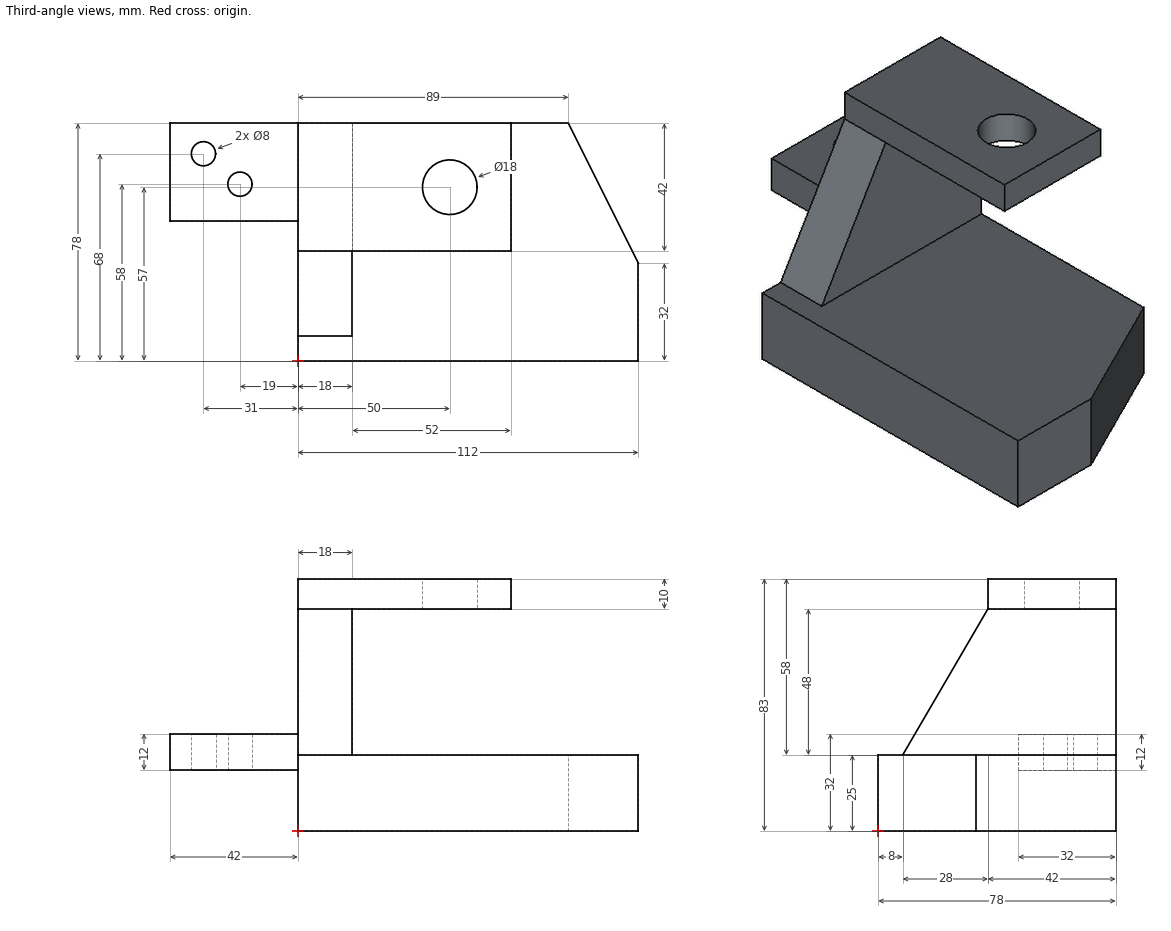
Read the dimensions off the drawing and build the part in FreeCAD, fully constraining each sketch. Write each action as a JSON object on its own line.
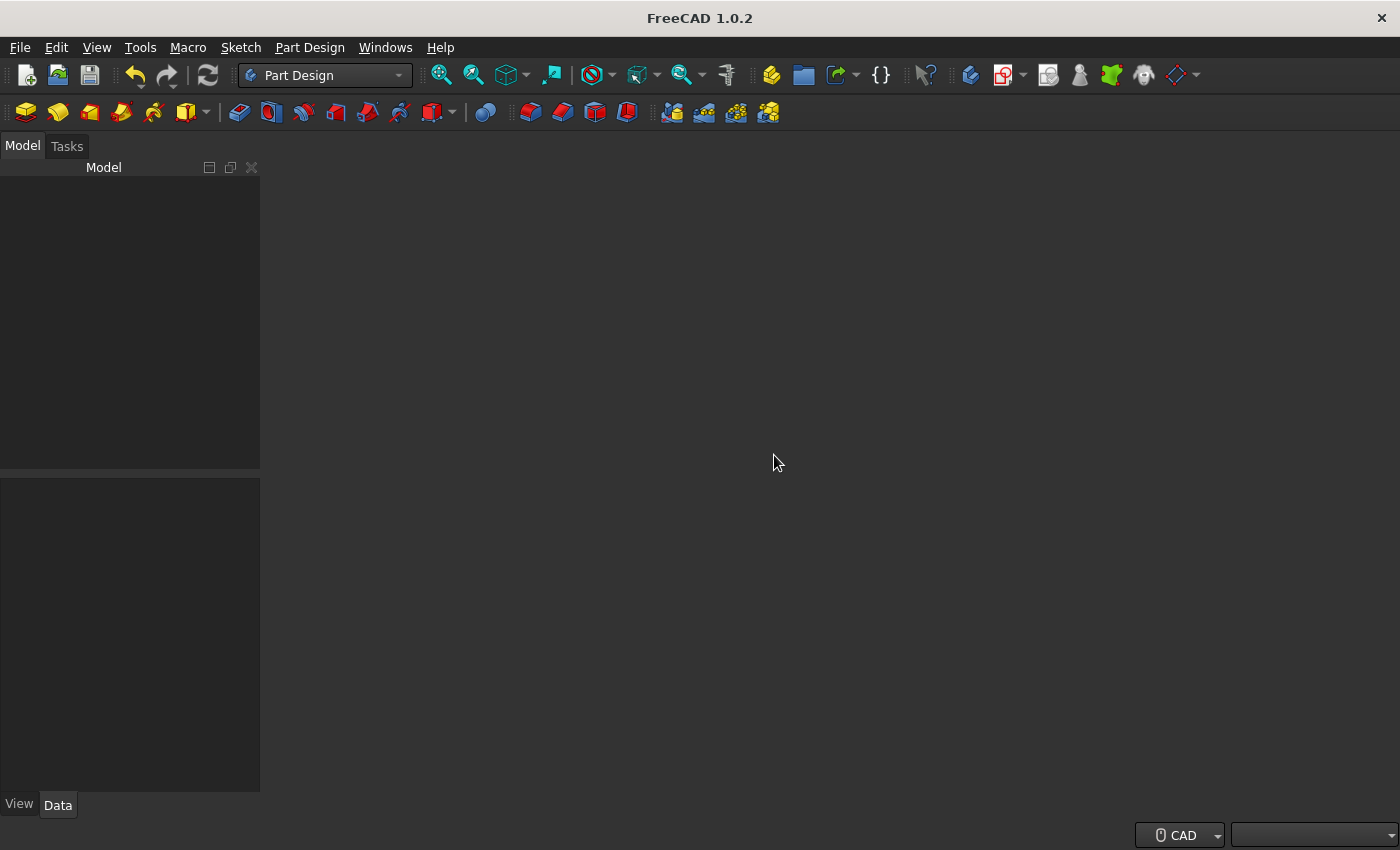
{"action": "key", "text": "ctrl+n"}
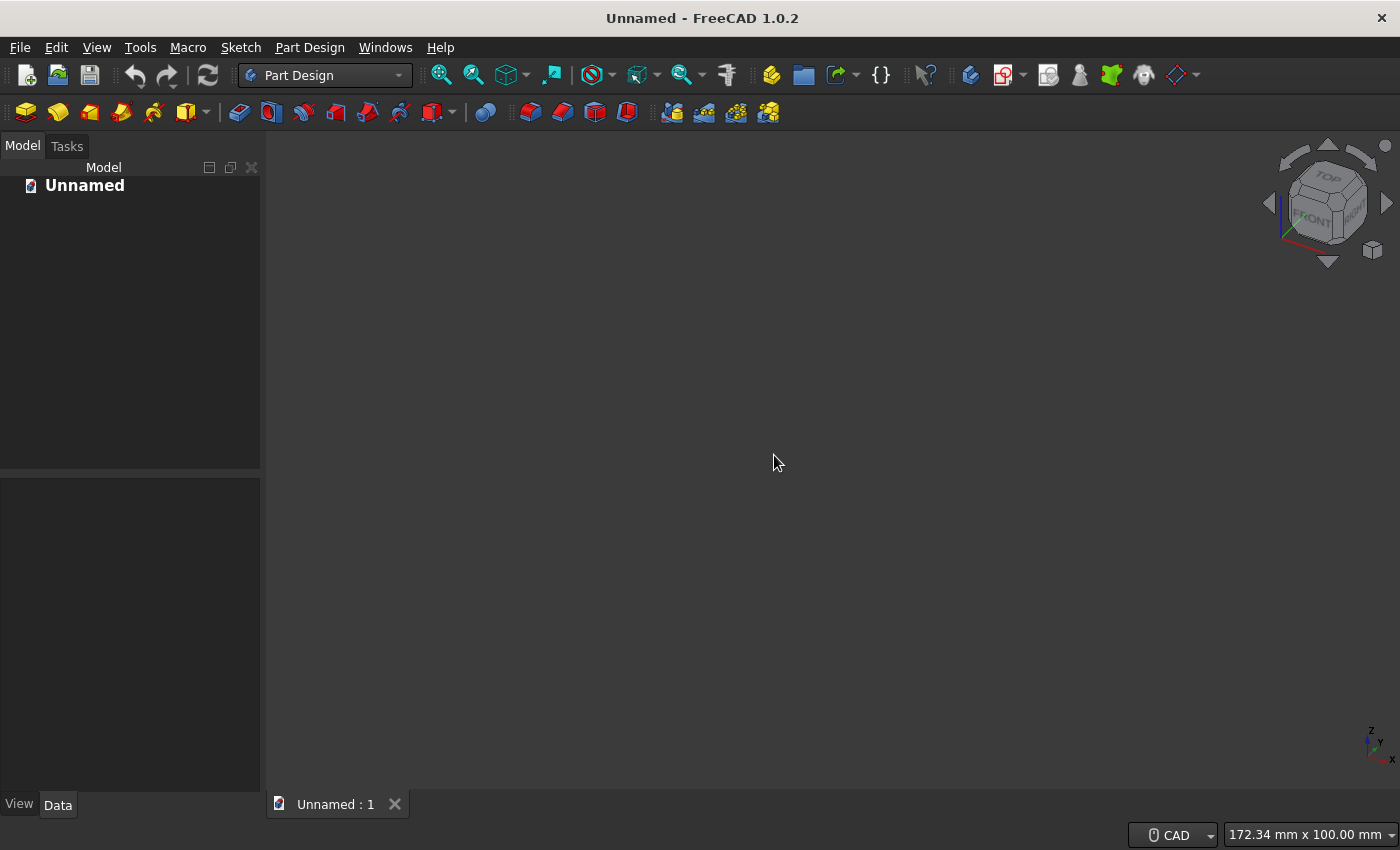
{"action": "left_click", "coordinate": [1004, 76]}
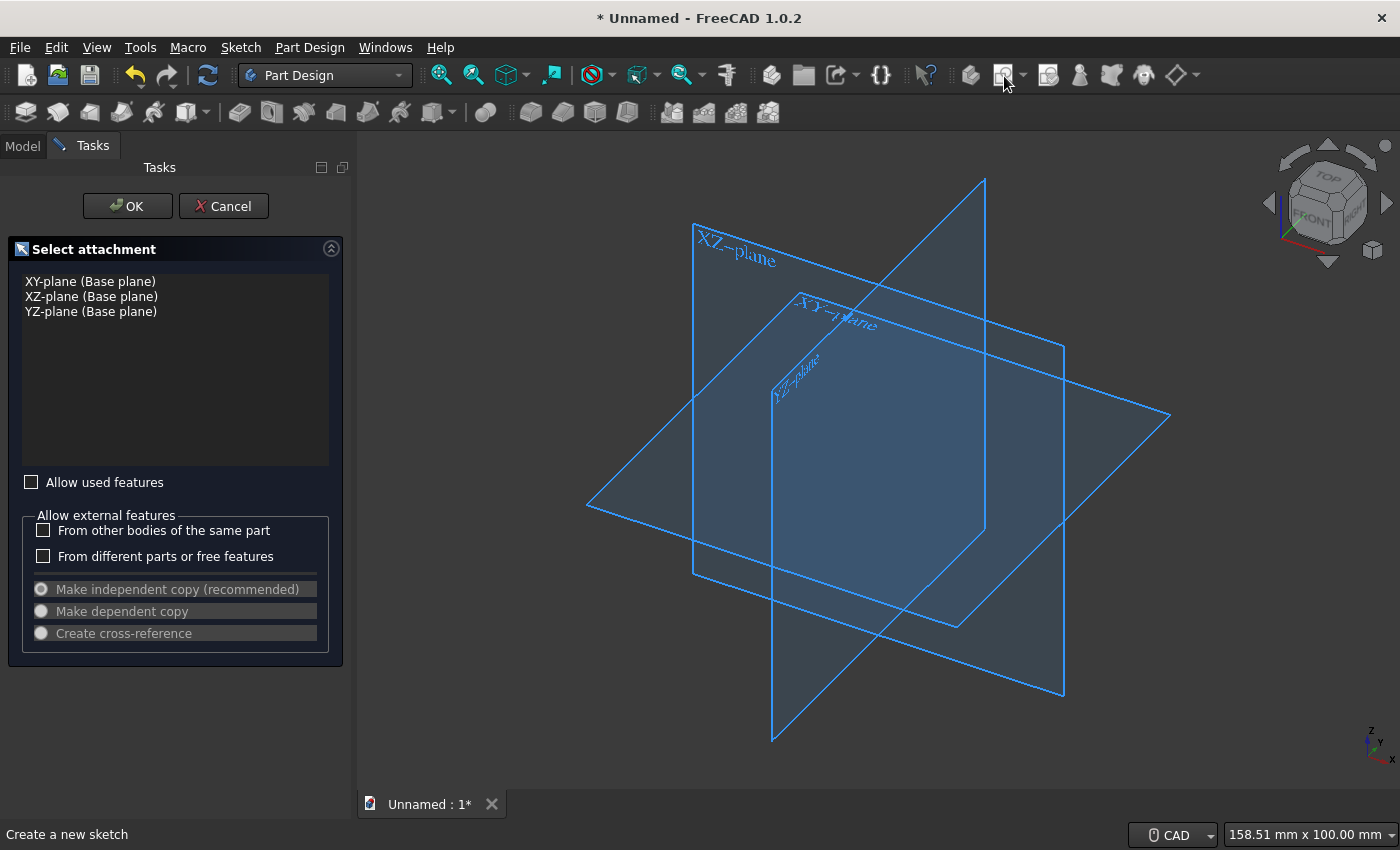
{"action": "left_click", "coordinate": [82, 282]}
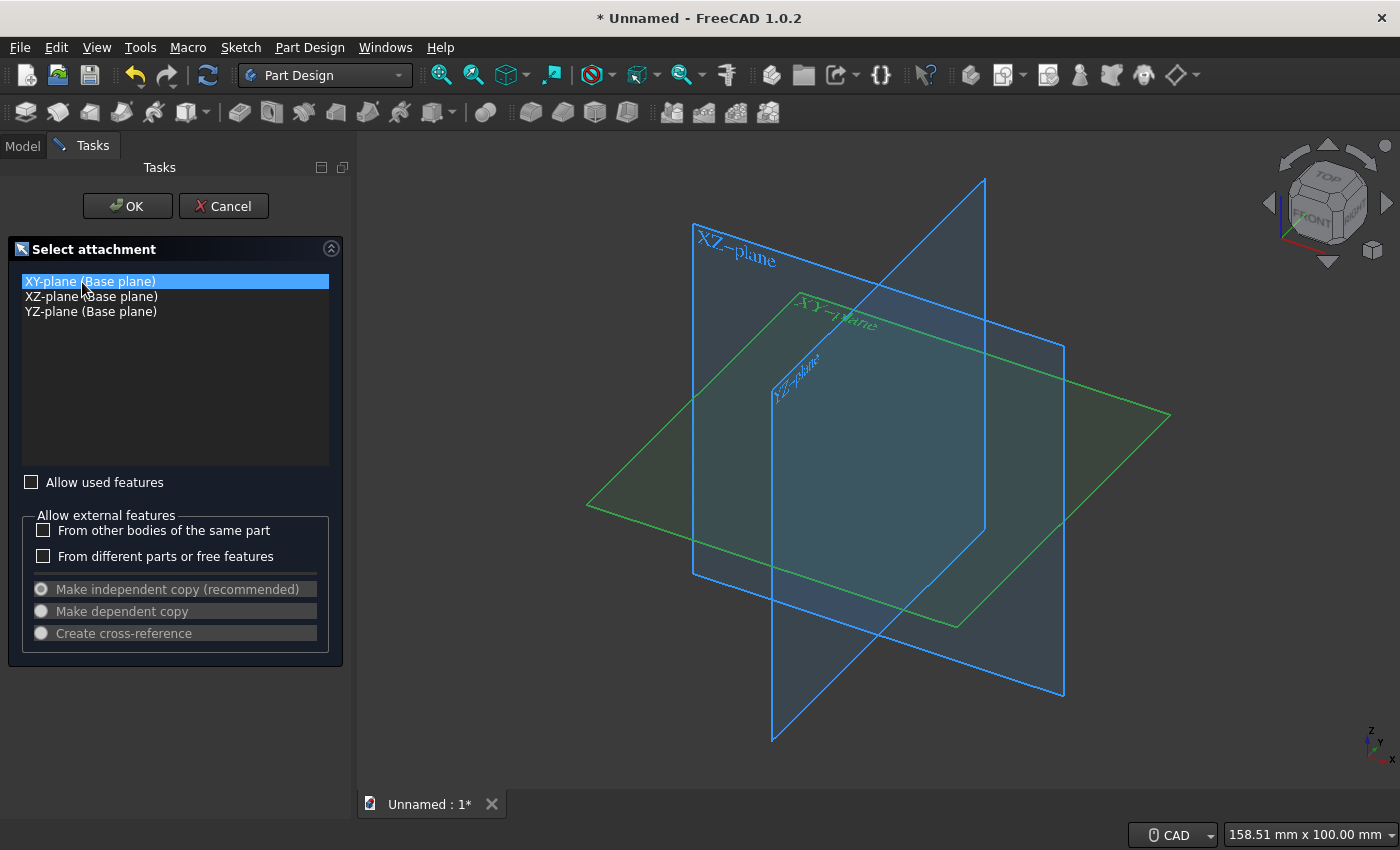
{"action": "left_click", "coordinate": [128, 206]}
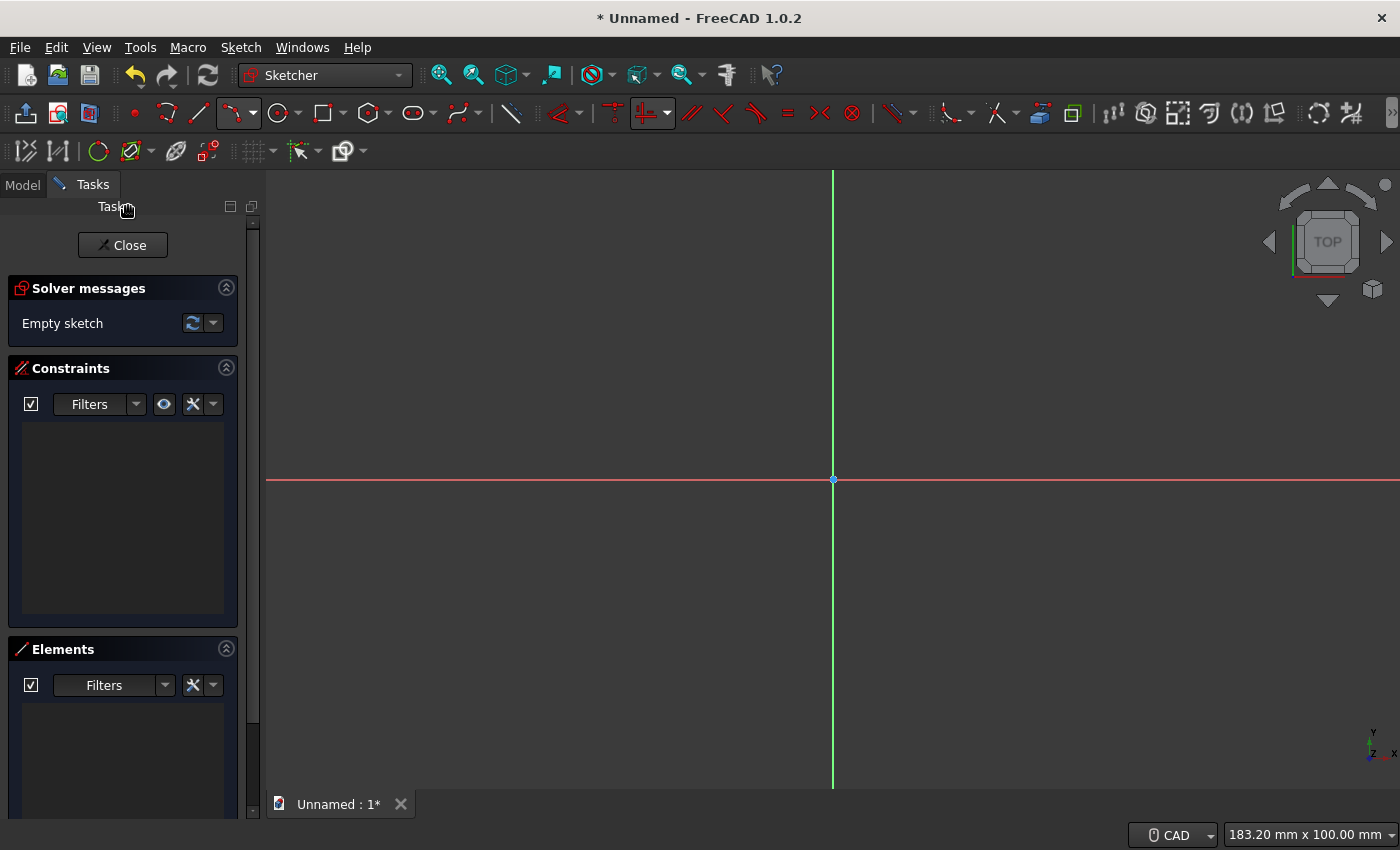
{"action": "scroll", "coordinate": [294, 761], "scroll_direction": "down", "scroll_amount": 2}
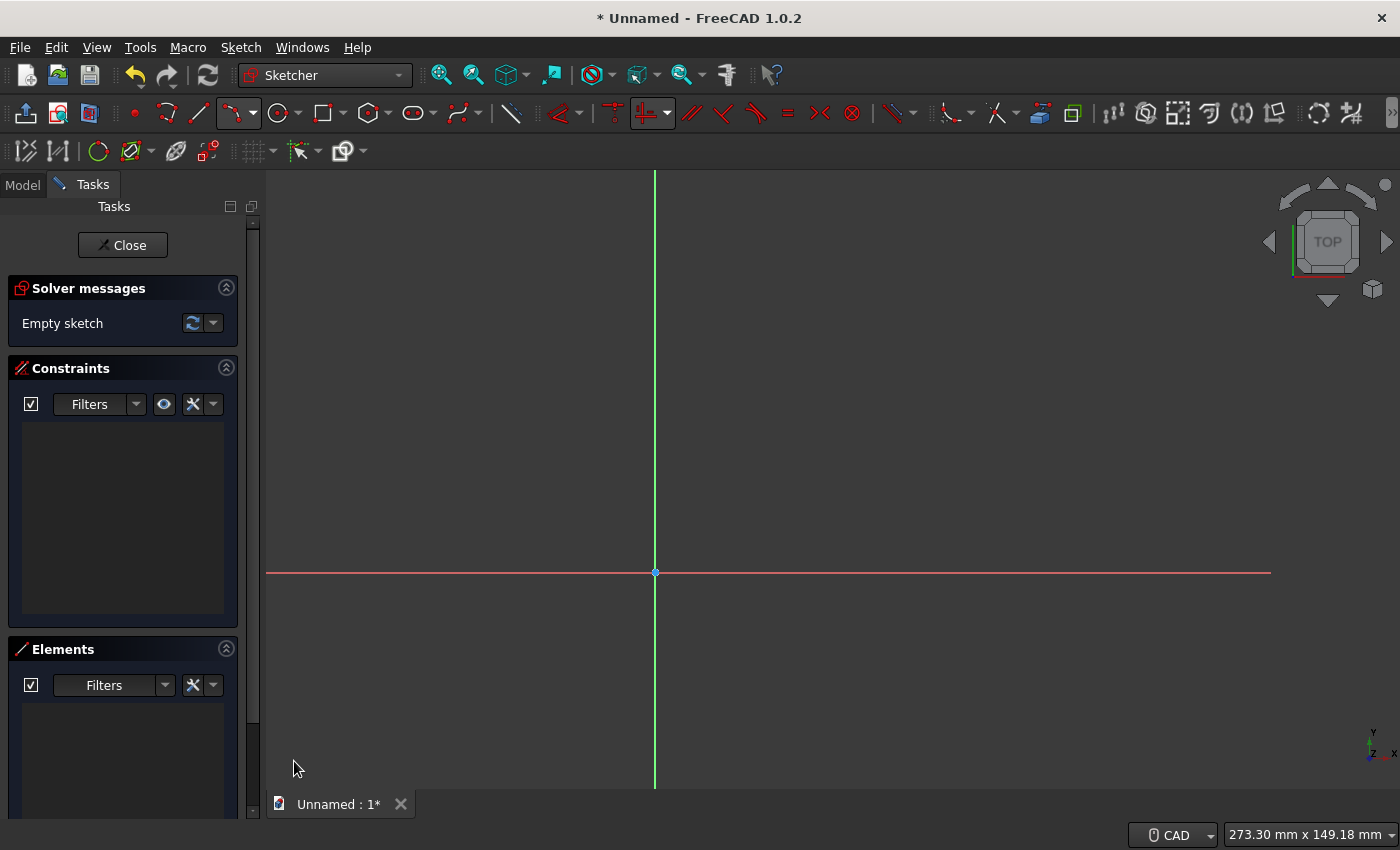
{"action": "key", "text": "g m"}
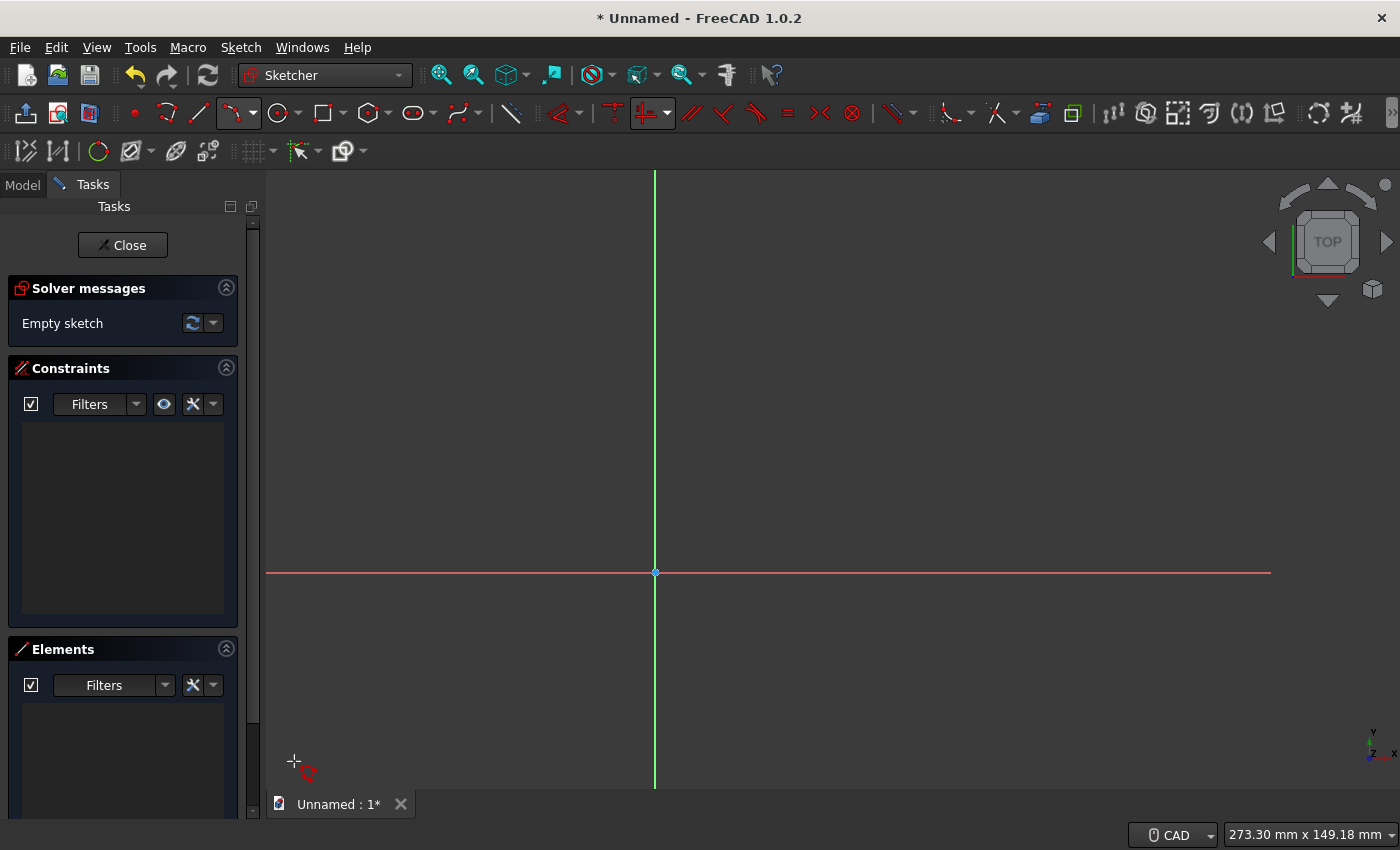
{"action": "left_click", "coordinate": [655, 573]}
{"action": "left_click", "coordinate": [1120, 564]}
{"action": "left_click", "coordinate": [1120, 440]}
{"action": "left_click", "coordinate": [1025, 249]}
{"action": "left_click", "coordinate": [664, 249]}
{"action": "left_click", "coordinate": [655, 573]}
{"action": "key", "text": "Escape"}
{"action": "key", "text": "Escape"}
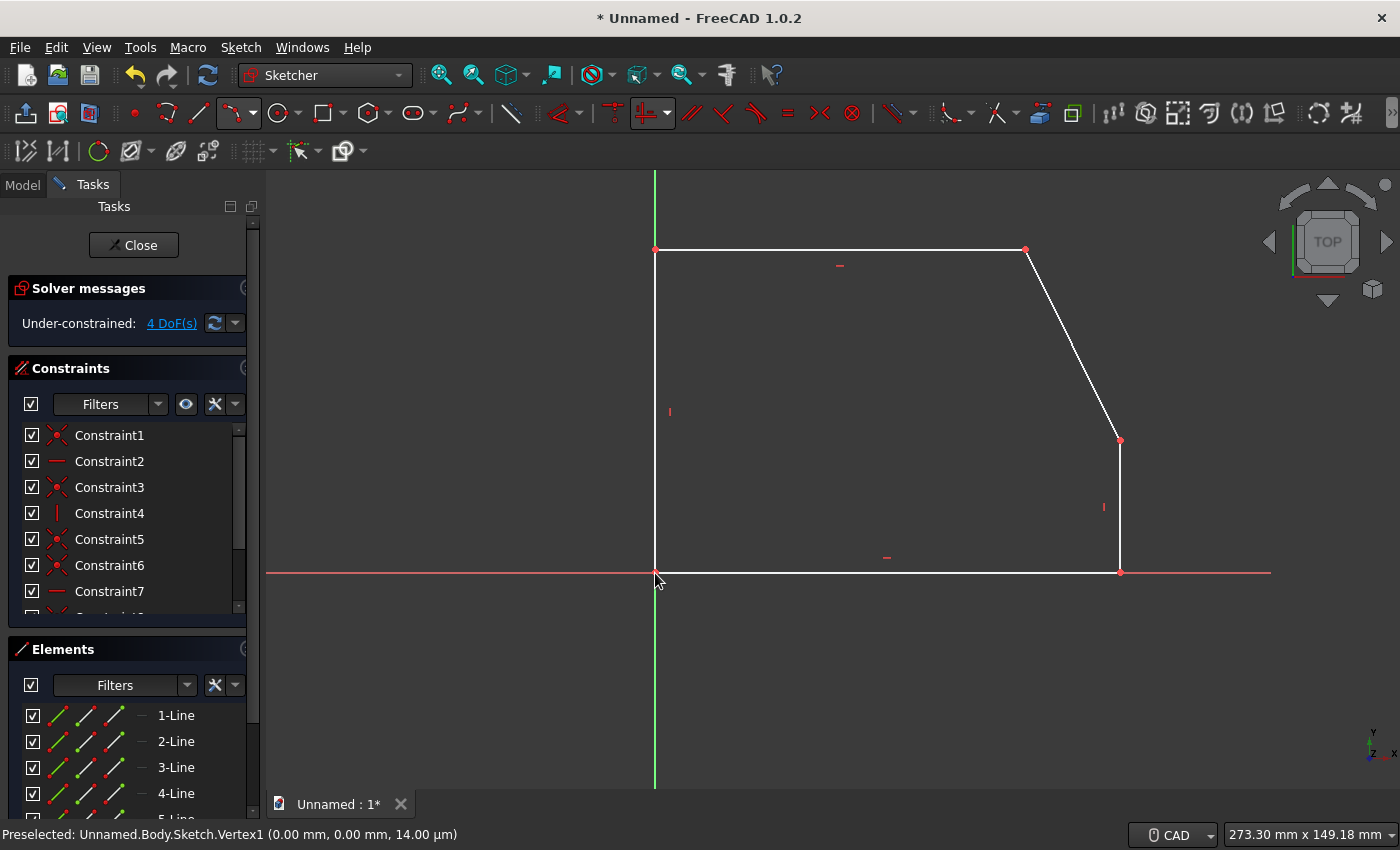
{"action": "left_click", "coordinate": [558, 114]}